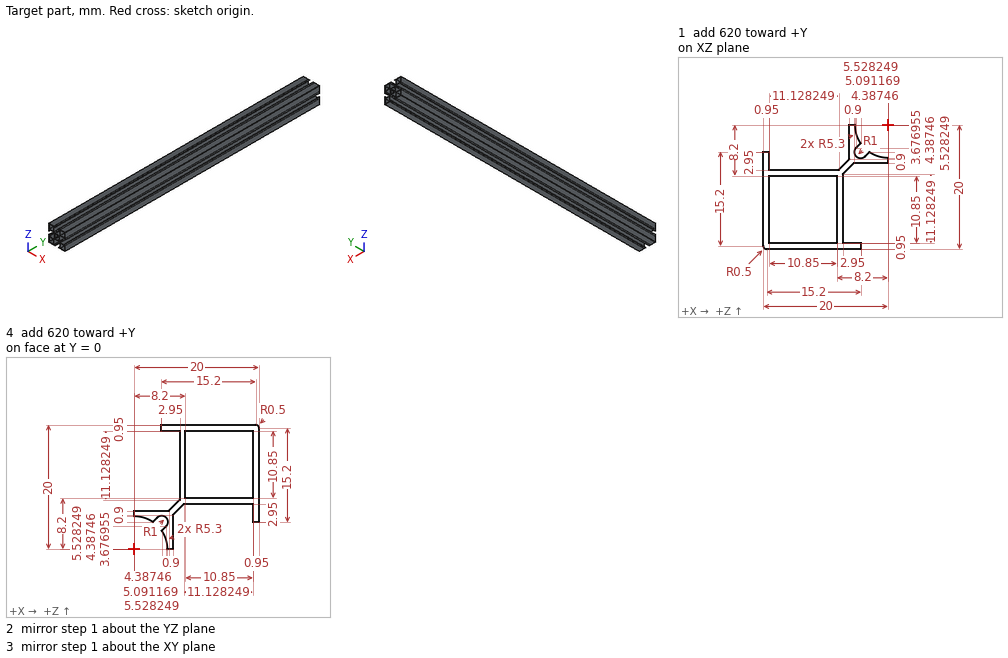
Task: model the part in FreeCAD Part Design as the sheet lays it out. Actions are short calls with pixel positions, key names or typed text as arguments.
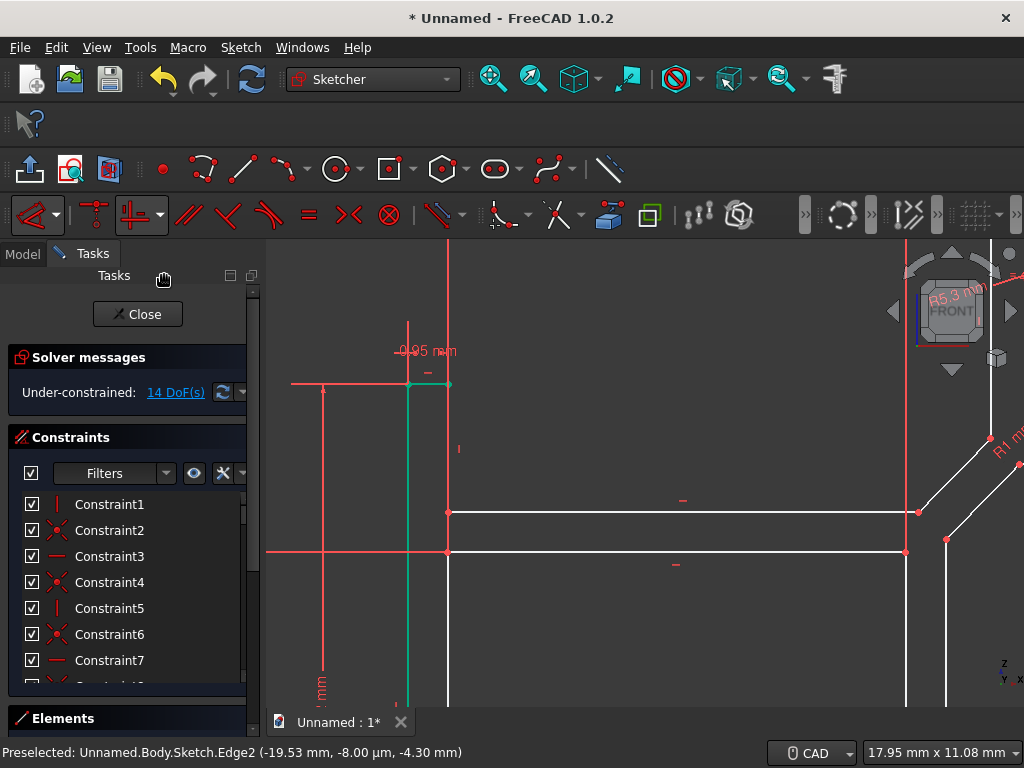
click(448, 423)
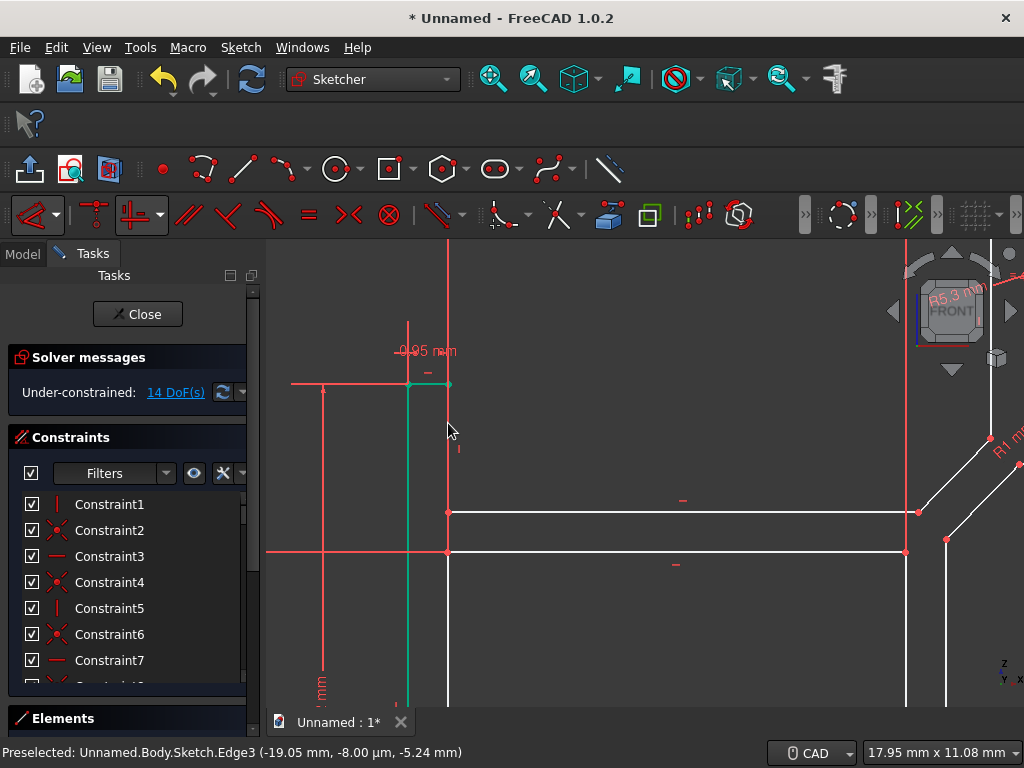
click(58, 216)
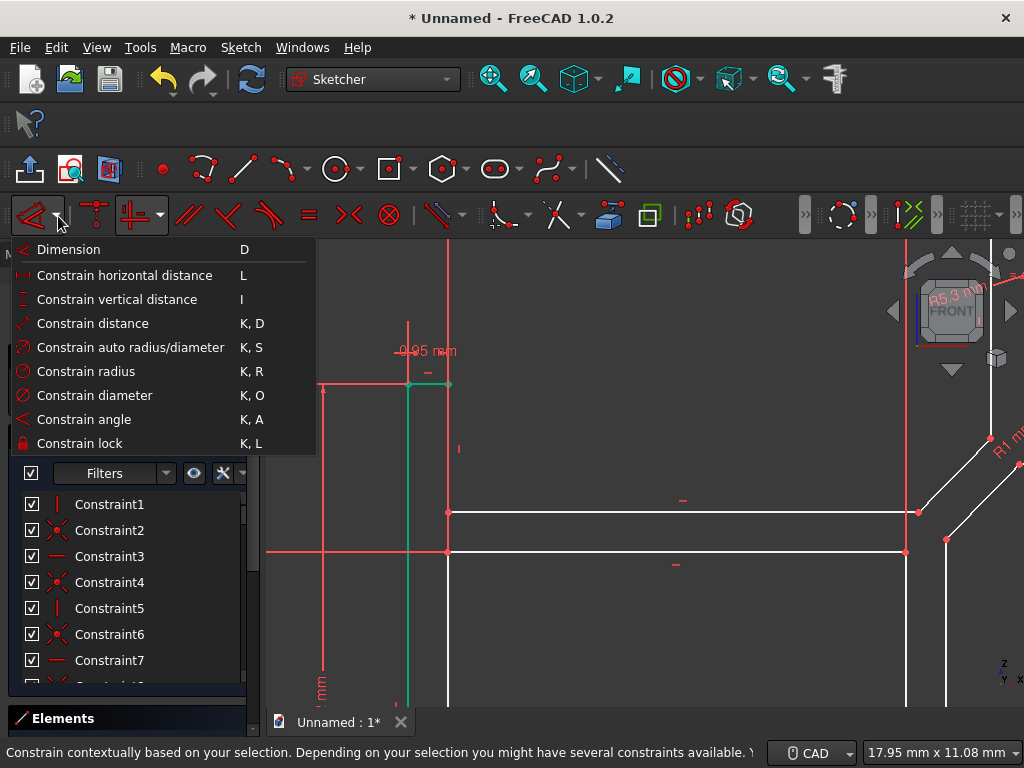
click(164, 299)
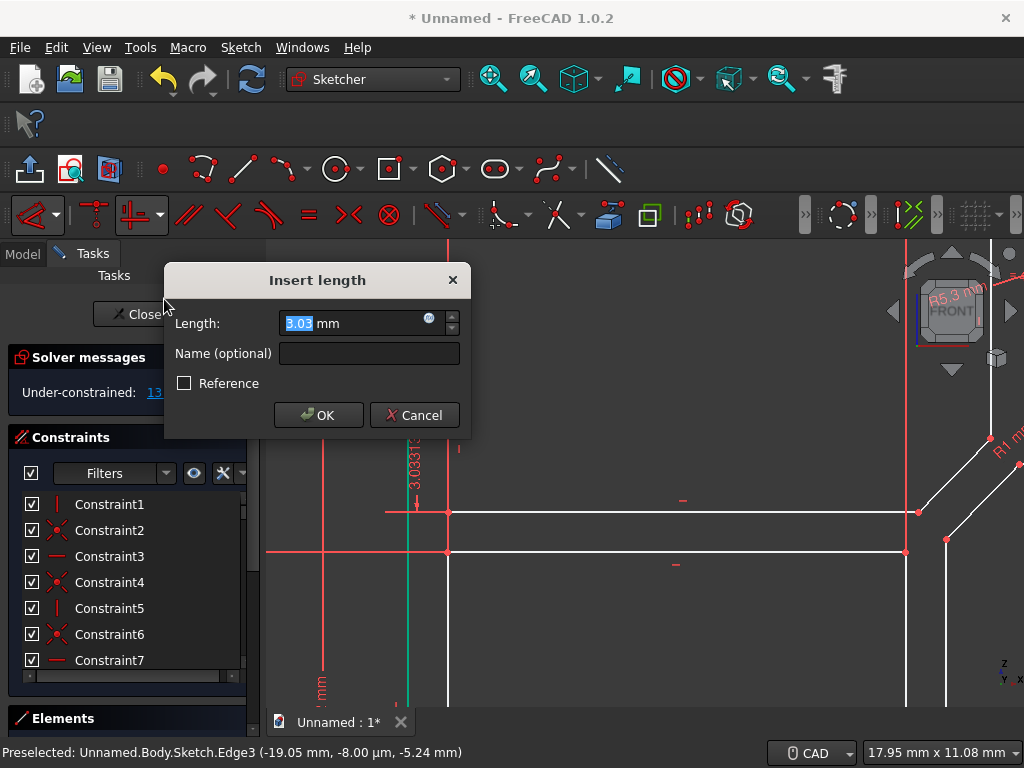
text(2.95)
key(Return)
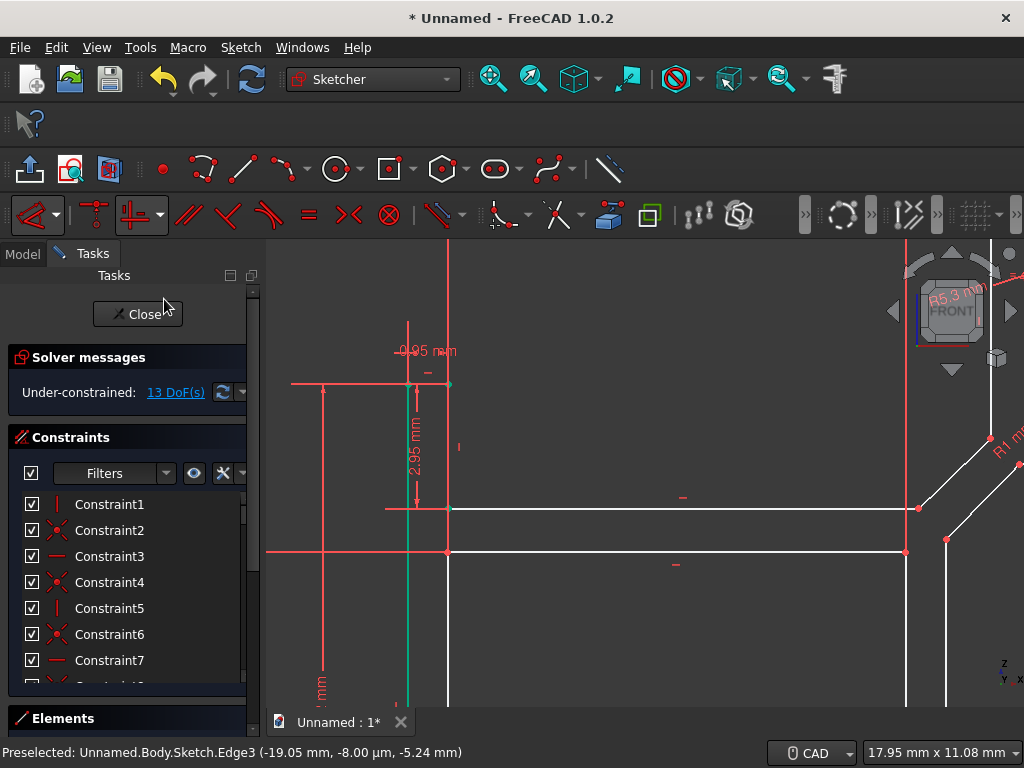
scroll(429, 385, down, 5)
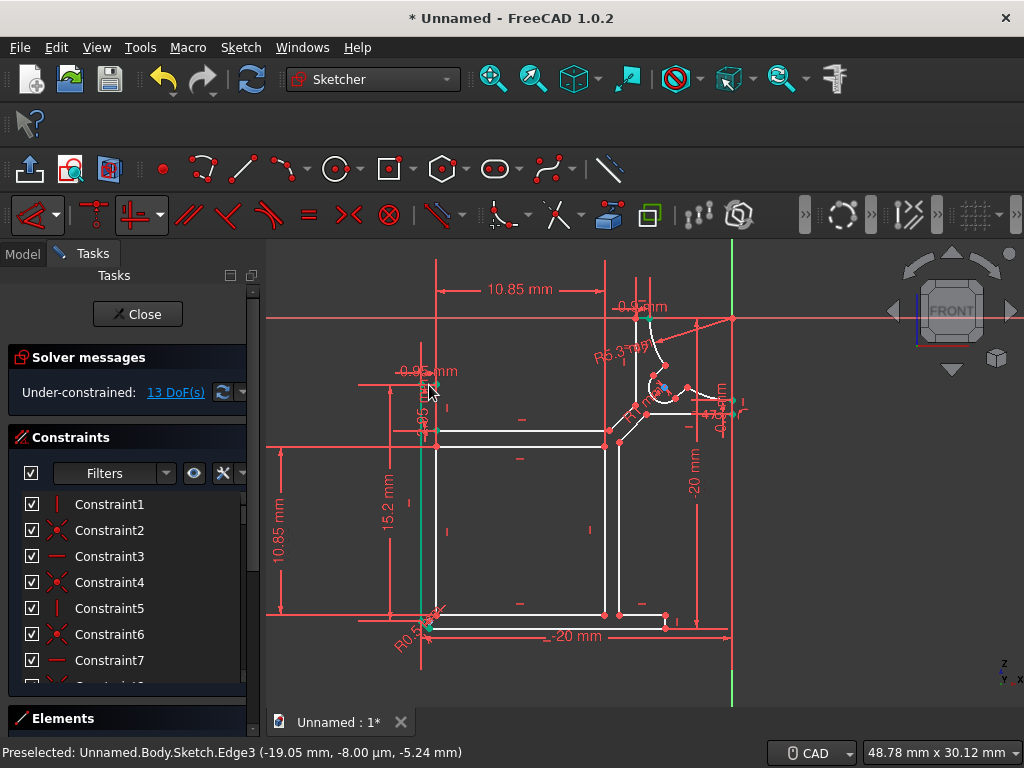
click(633, 615)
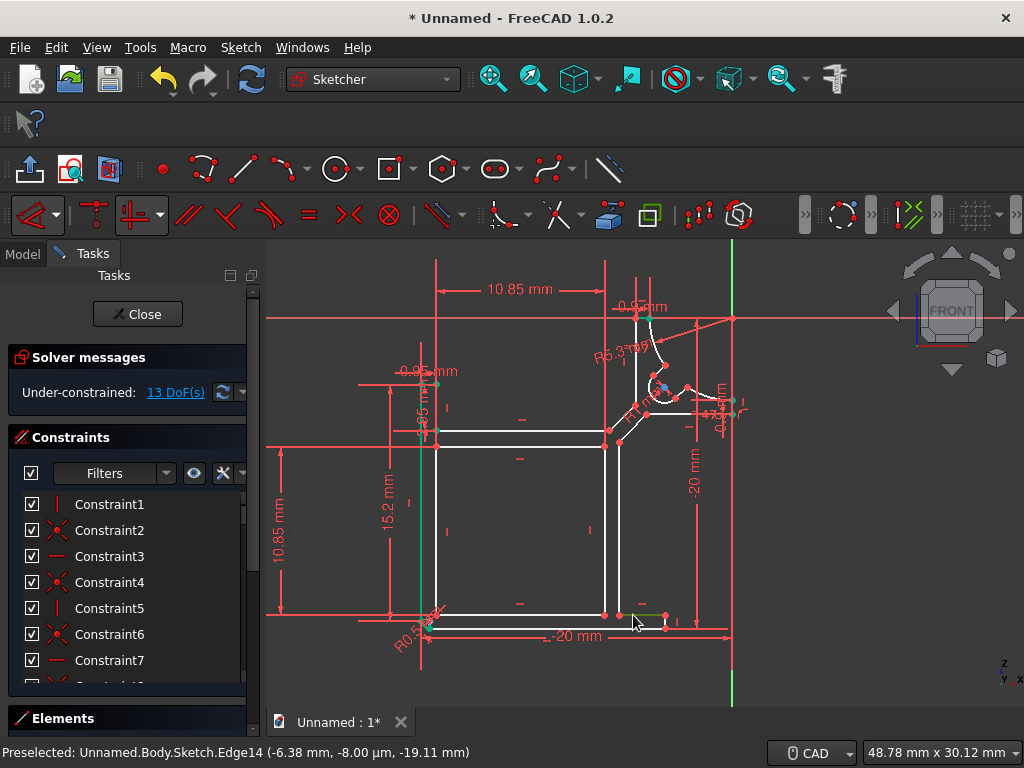
click(58, 216)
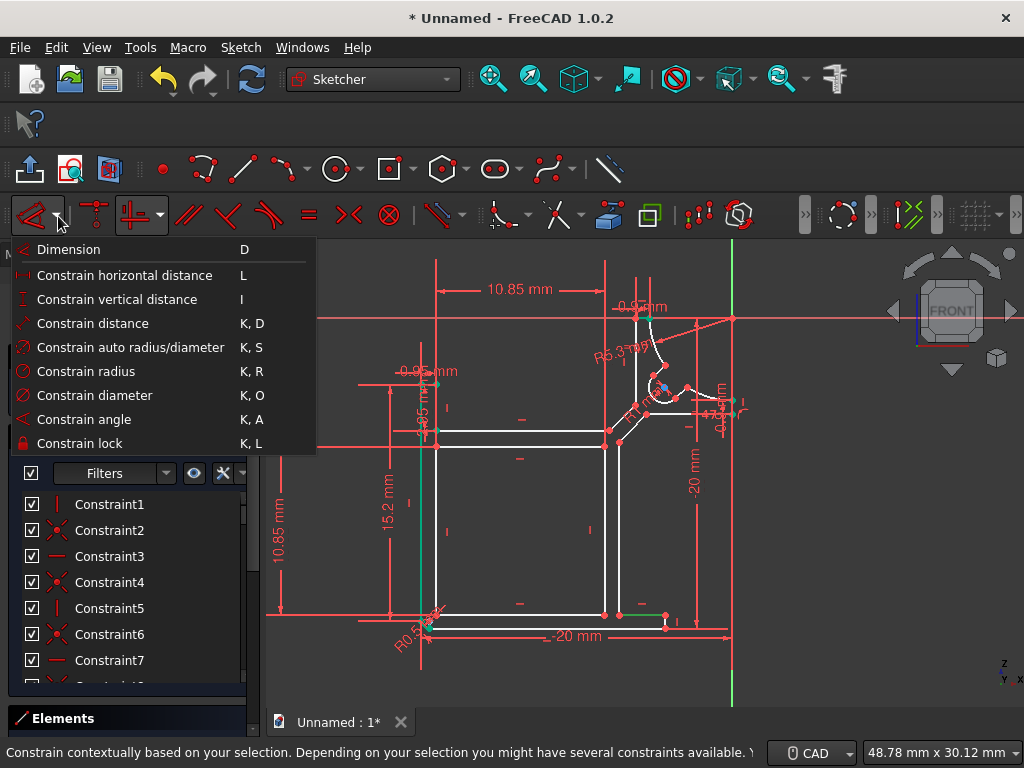
click(164, 275)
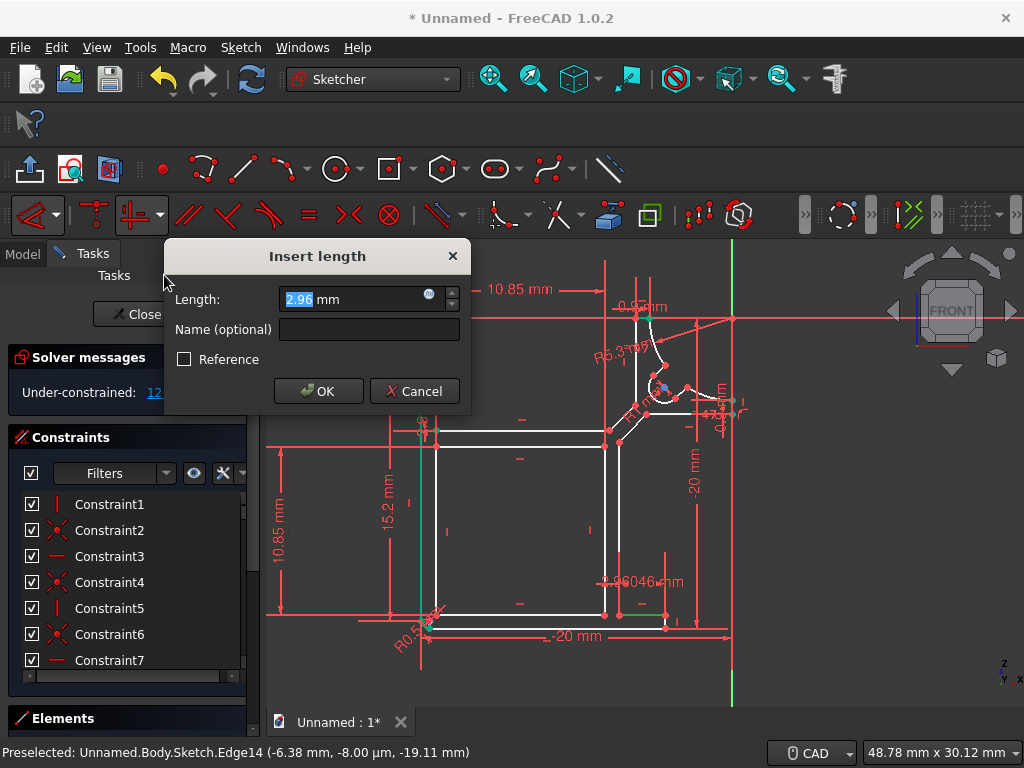
text(2.95)
key(Return)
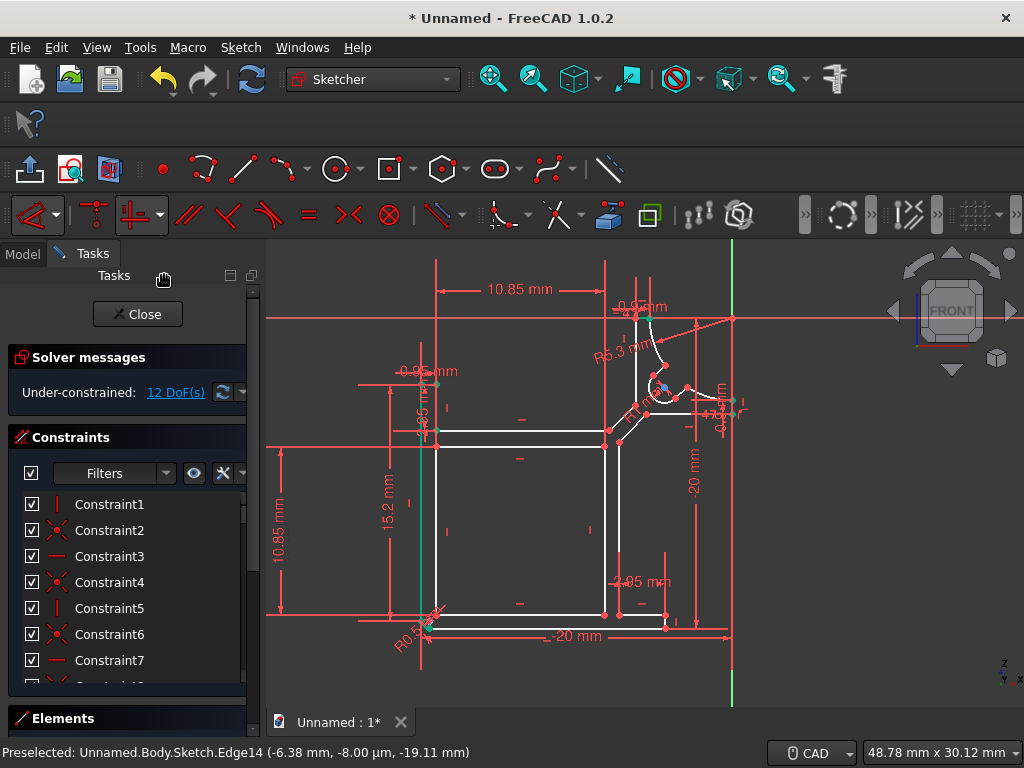
scroll(665, 622, up, 5)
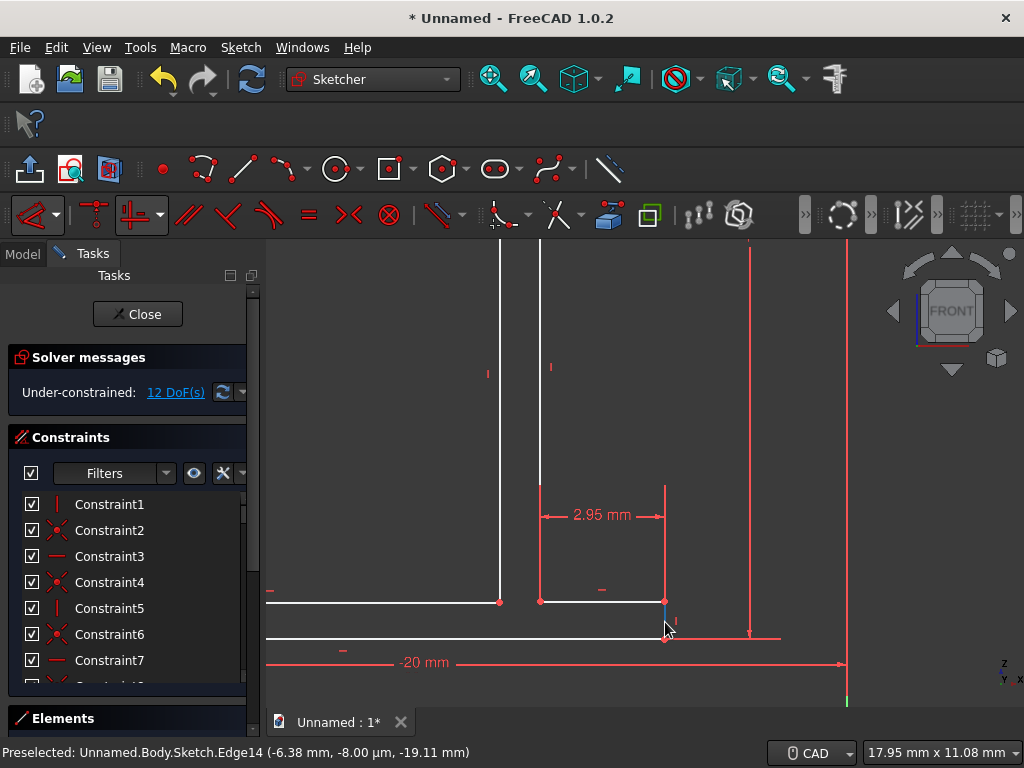
click(665, 620)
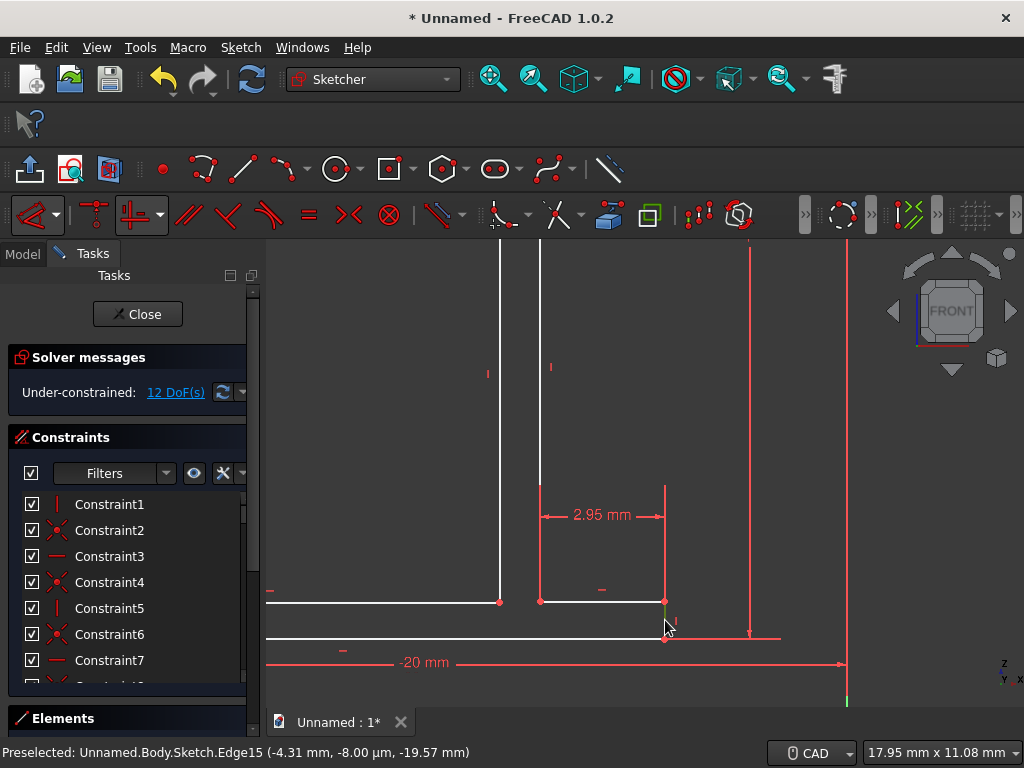
click(58, 216)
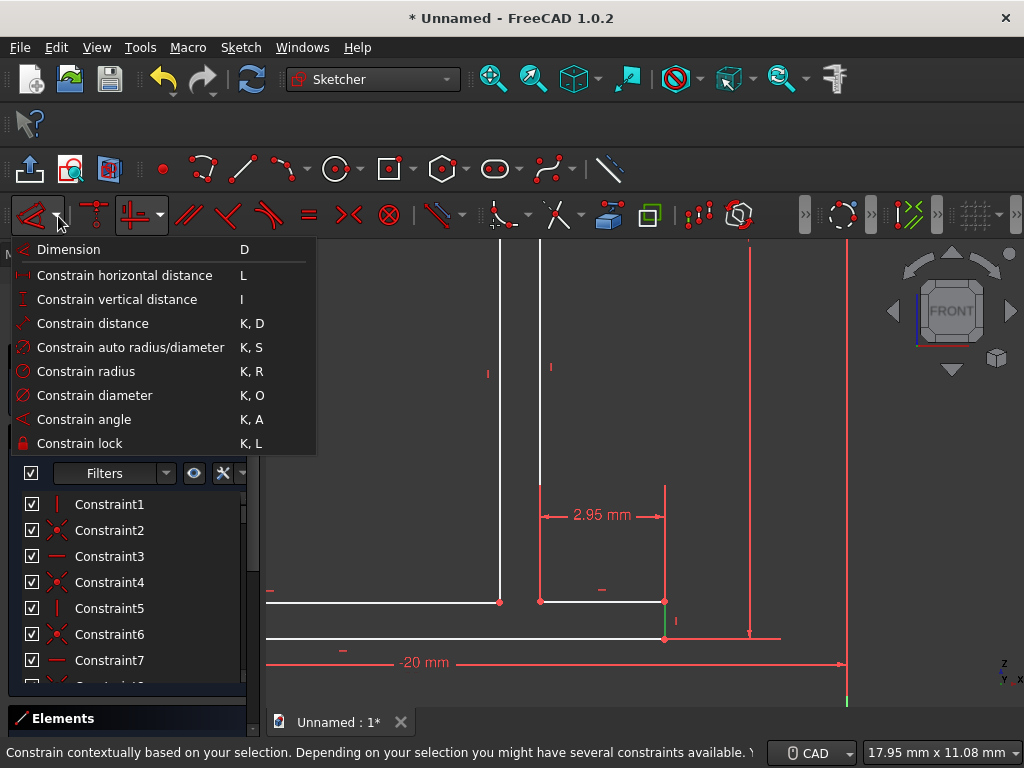
click(164, 299)